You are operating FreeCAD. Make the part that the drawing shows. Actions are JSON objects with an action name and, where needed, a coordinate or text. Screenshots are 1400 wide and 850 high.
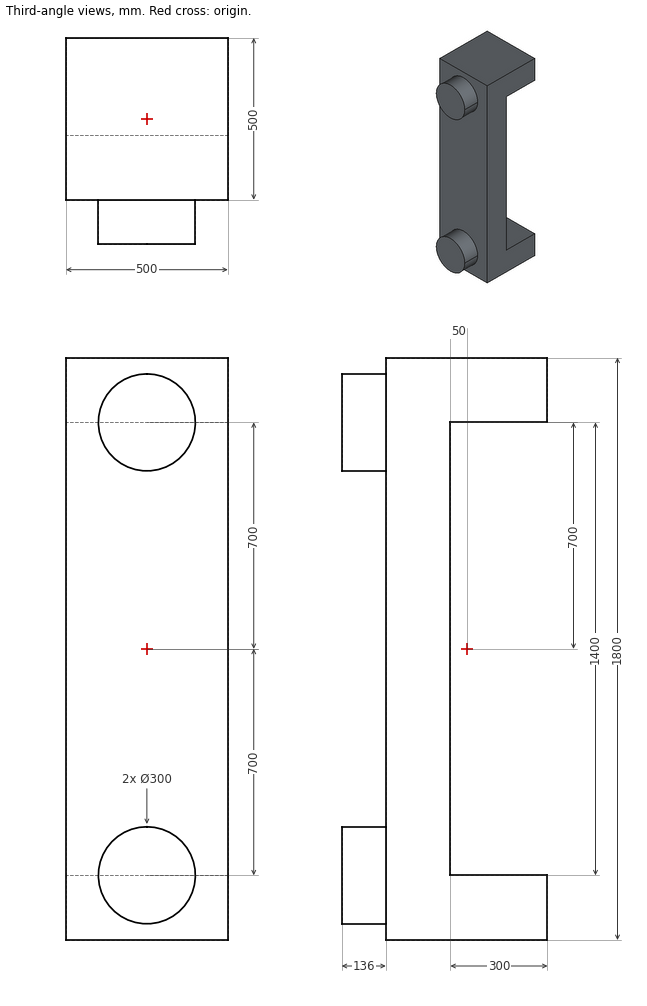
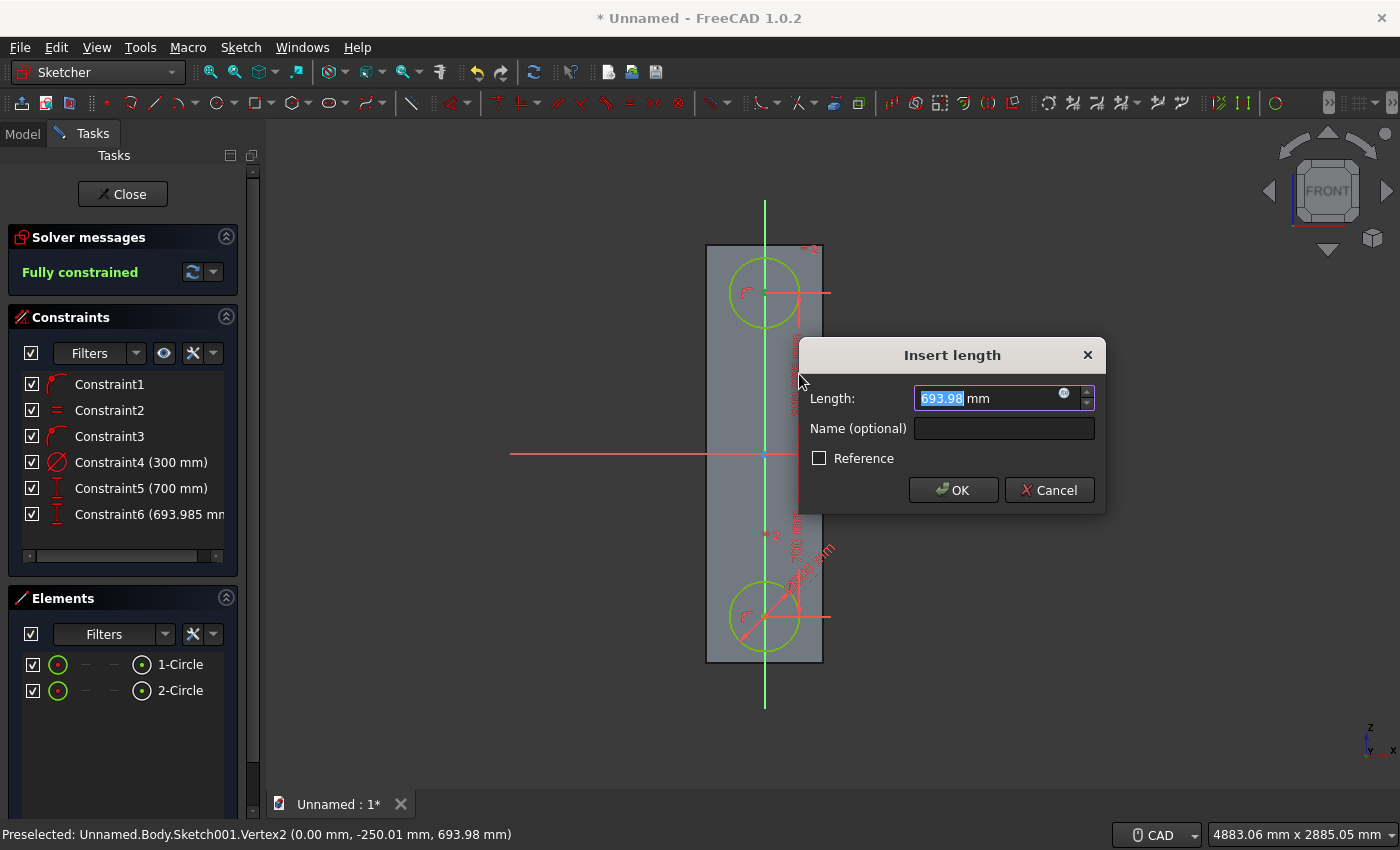
{"action": "type", "text": "700"}
{"action": "key", "text": "Return"}
{"action": "key", "text": "Escape"}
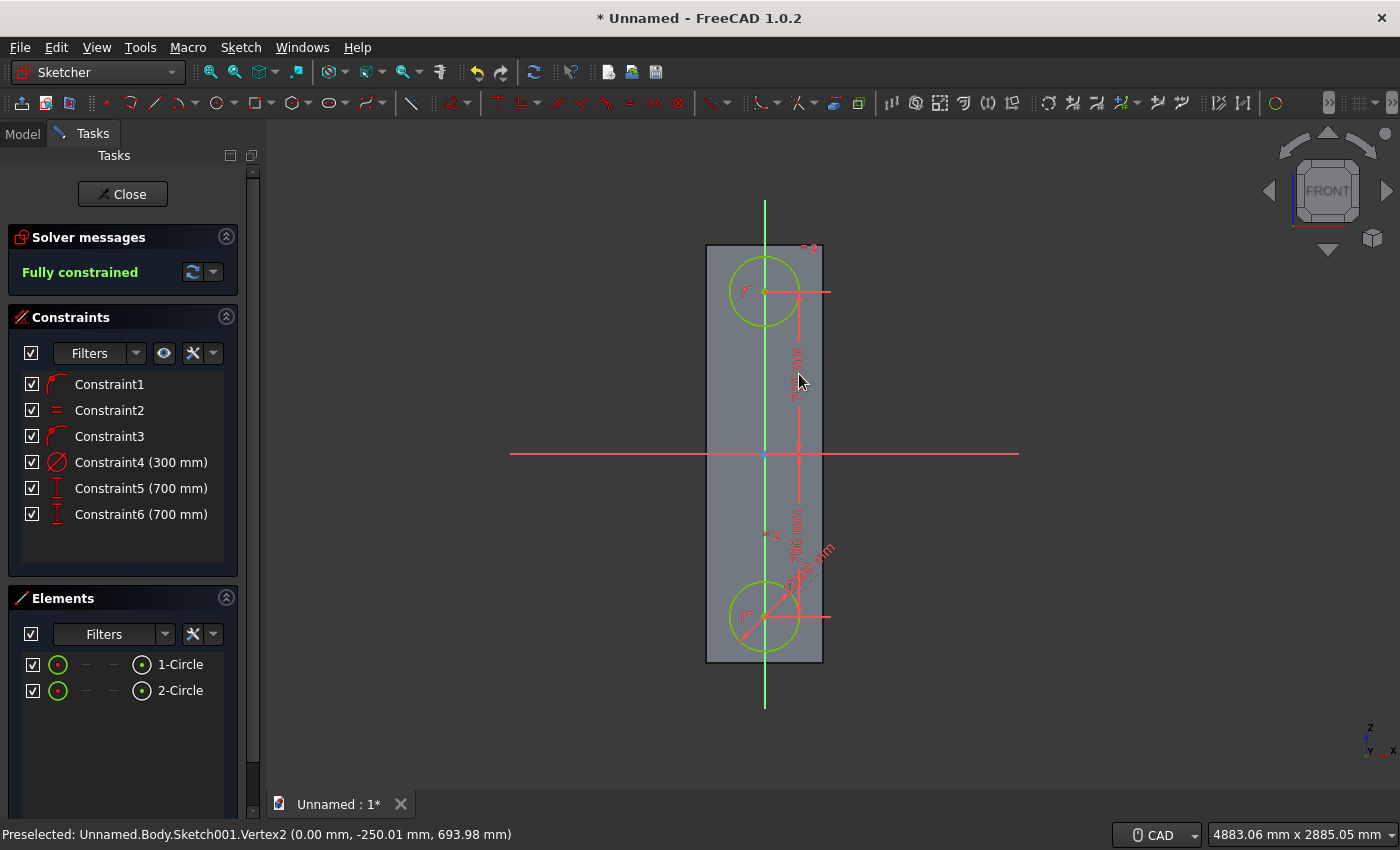
{"action": "left_click", "coordinate": [123, 194]}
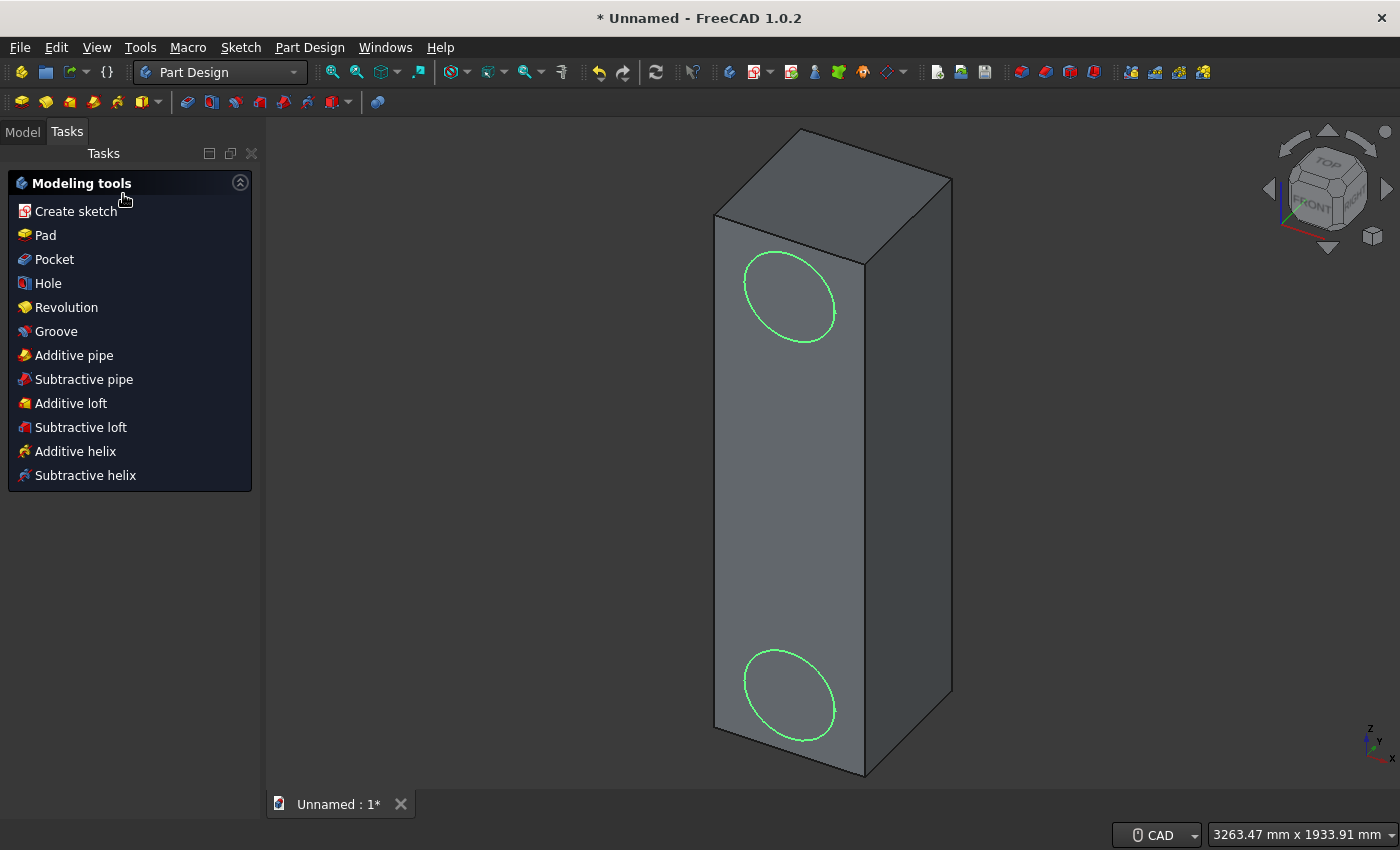
{"action": "left_click", "coordinate": [22, 102]}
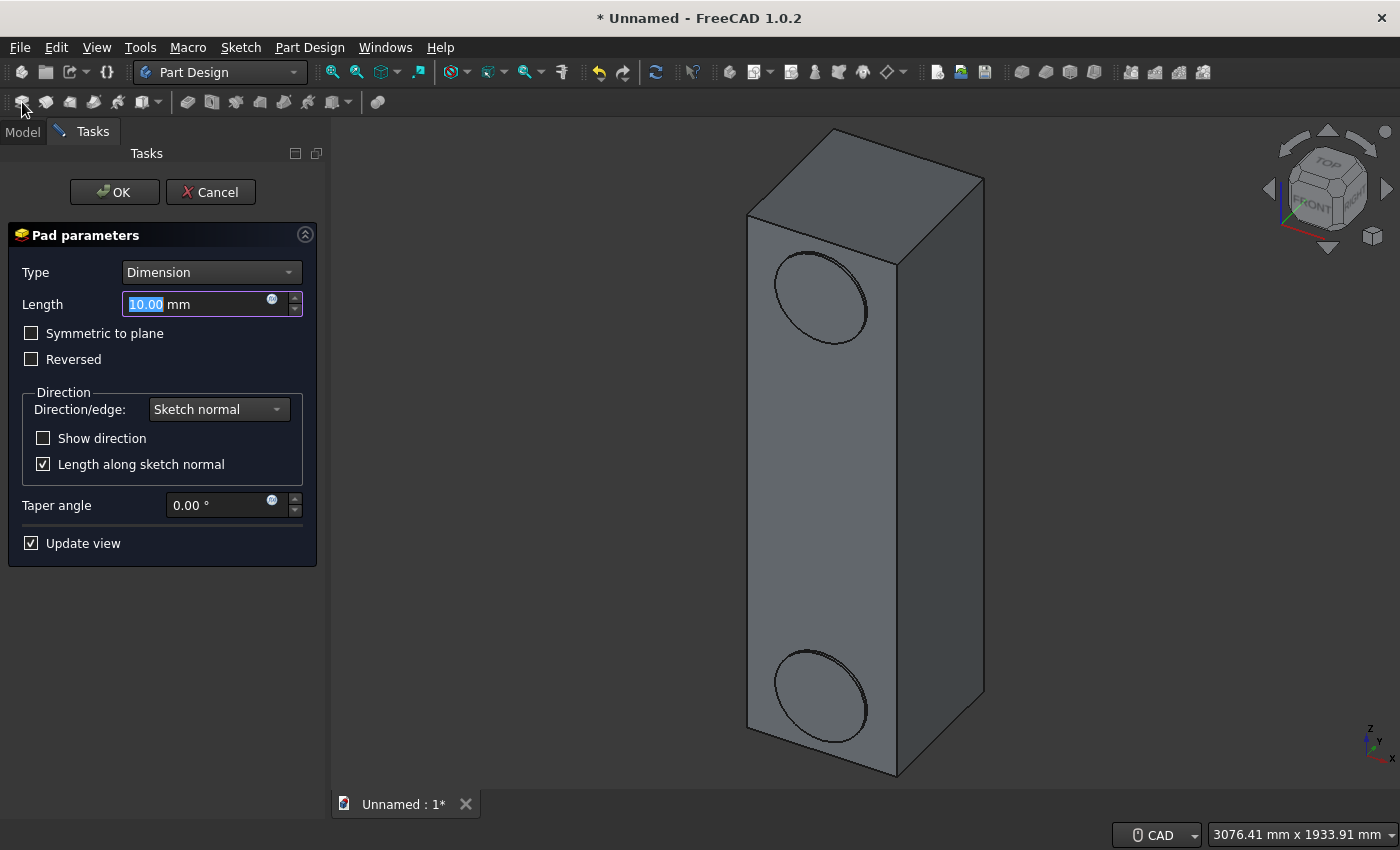
{"action": "type", "text": "136"}
{"action": "key", "text": "Tab"}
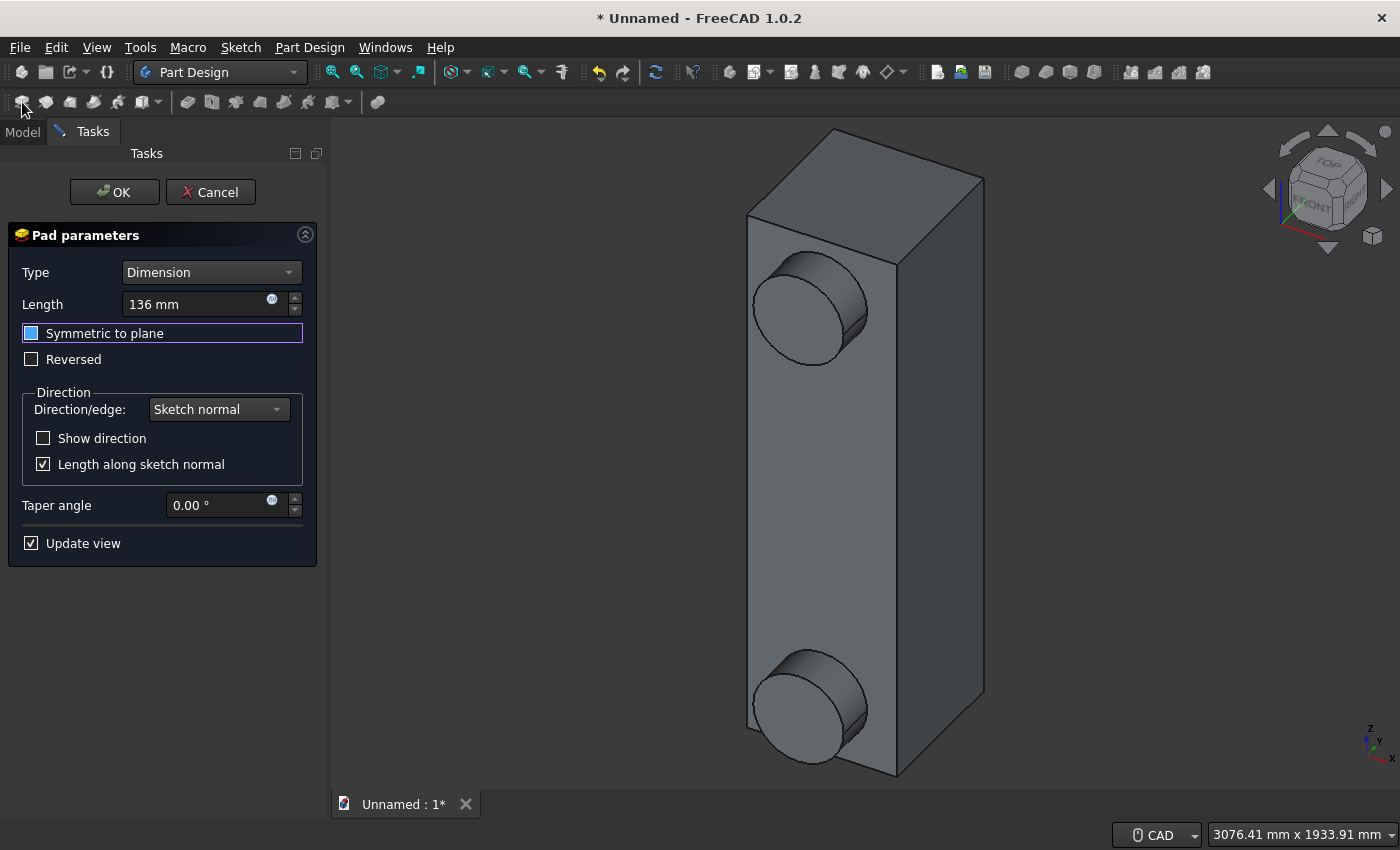
{"action": "left_click", "coordinate": [115, 192]}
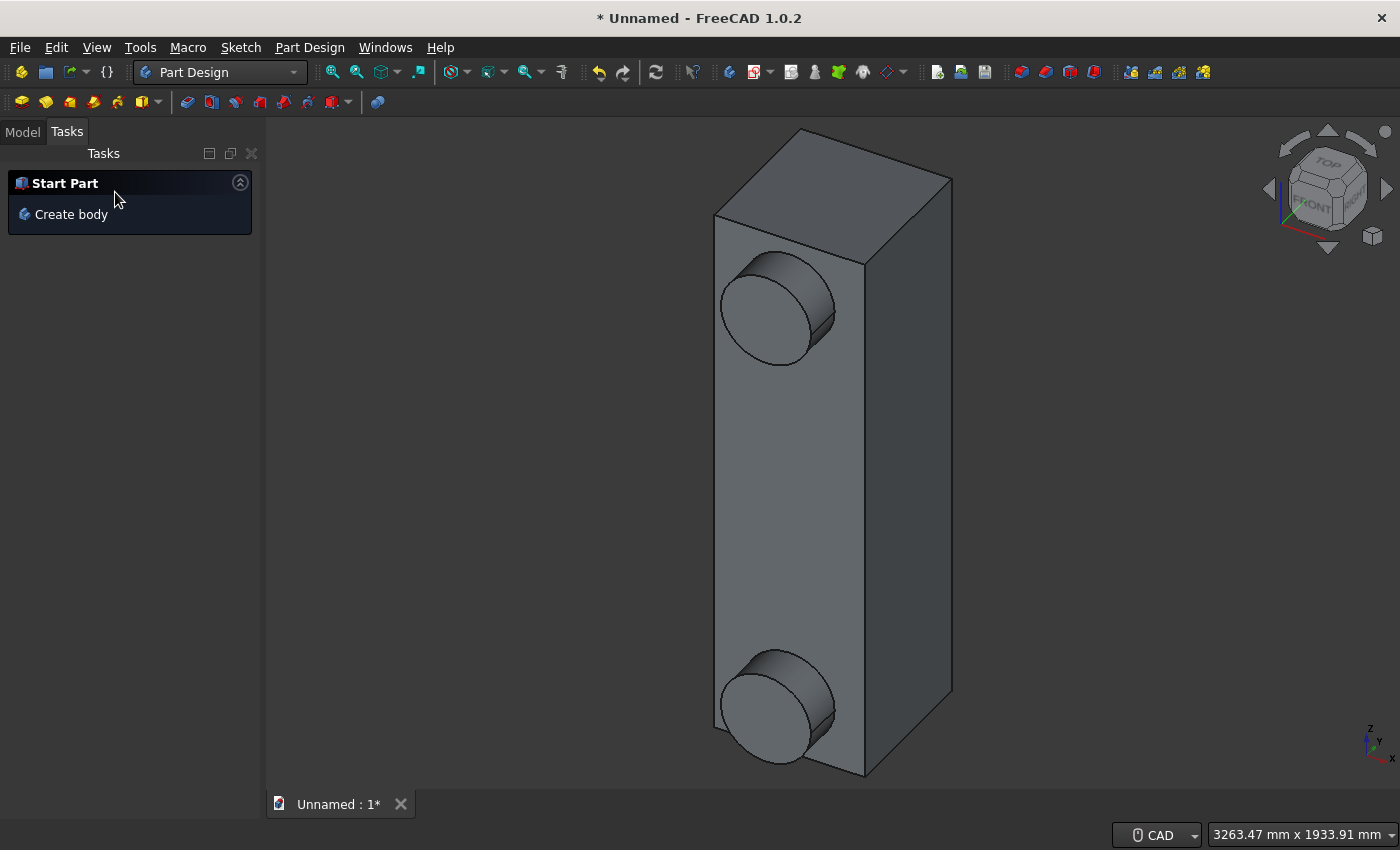
{"action": "left_click", "coordinate": [334, 72]}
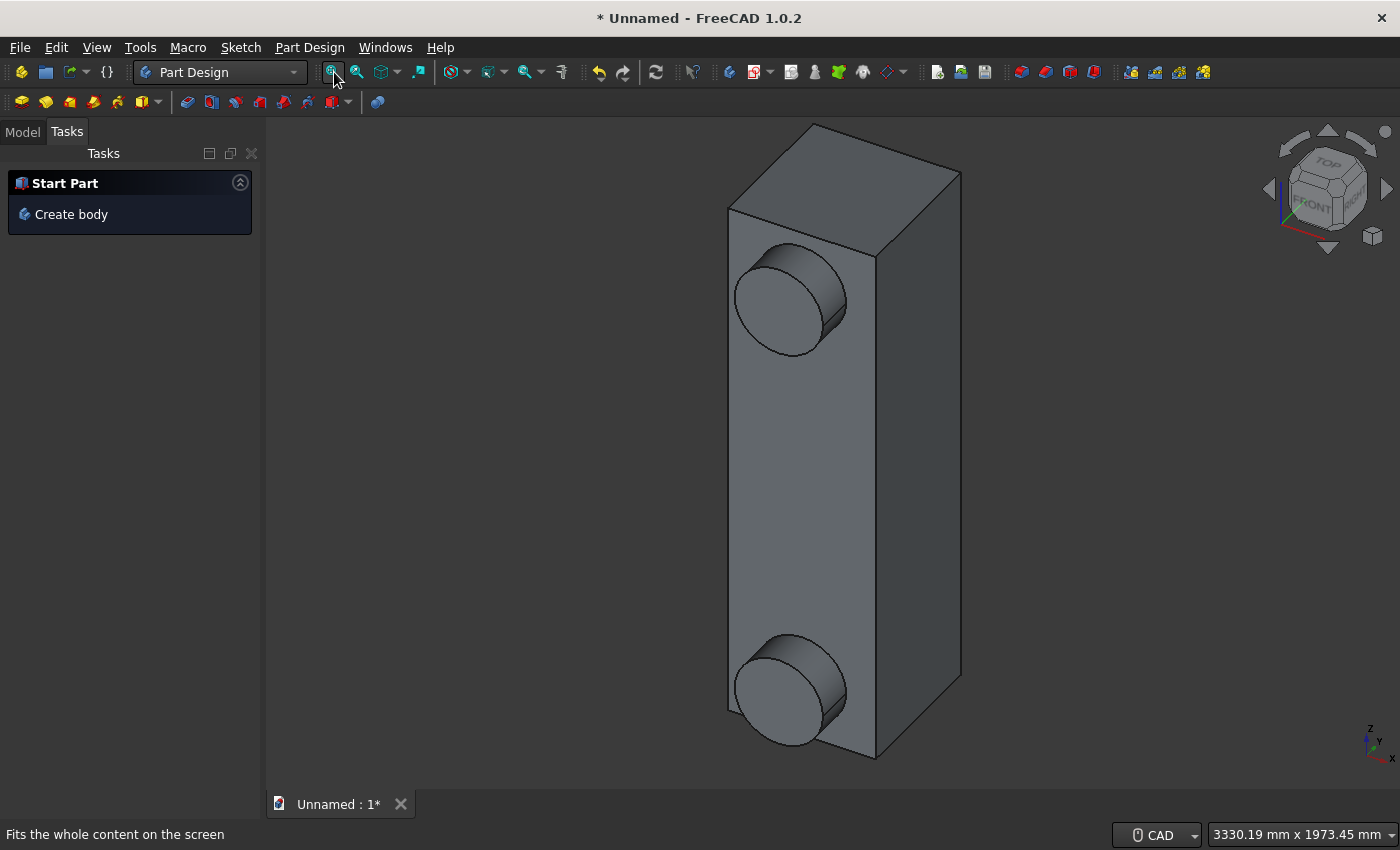
{"action": "left_click", "coordinate": [918, 321]}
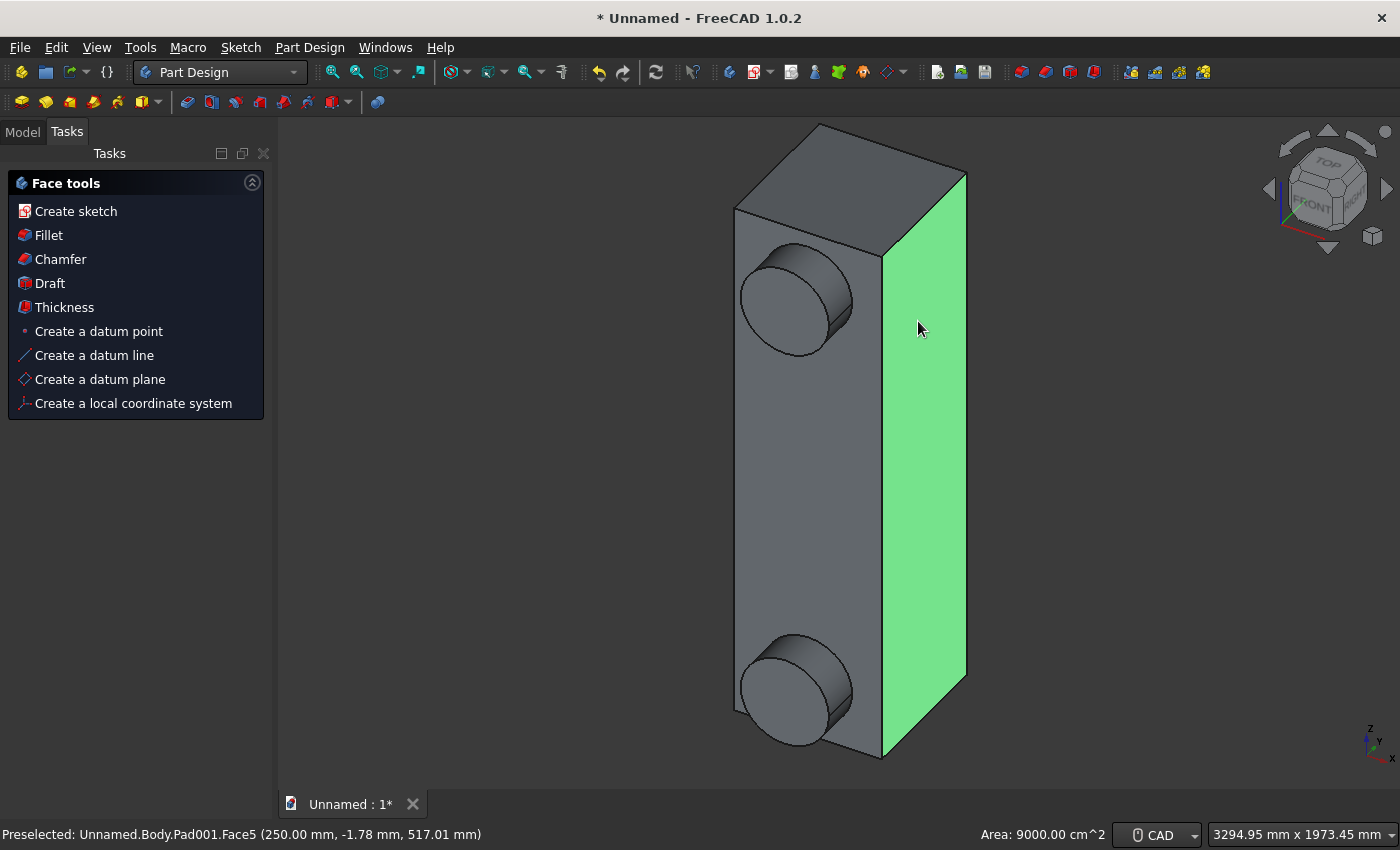
{"action": "left_click", "coordinate": [754, 72]}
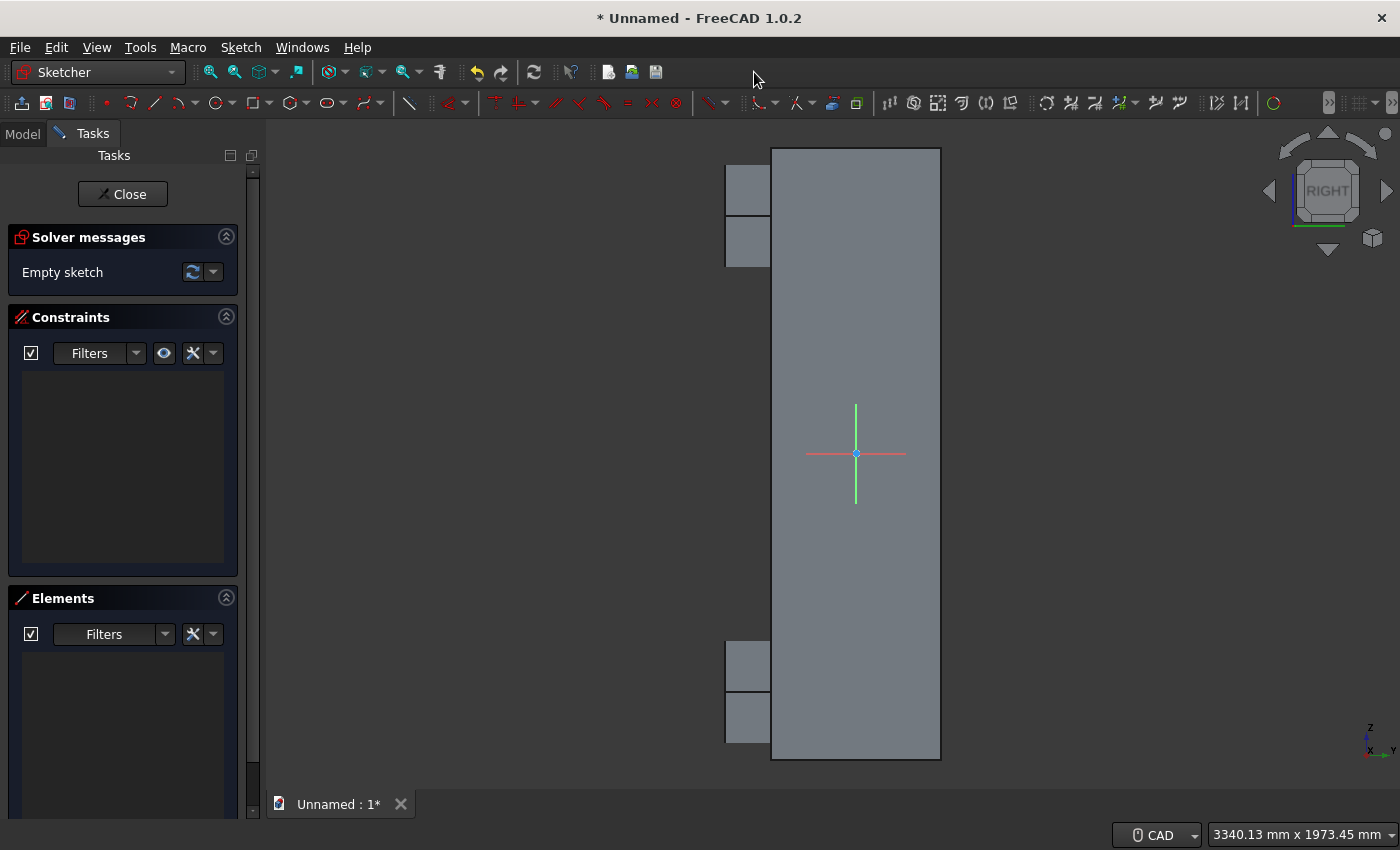
{"action": "left_click", "coordinate": [254, 104]}